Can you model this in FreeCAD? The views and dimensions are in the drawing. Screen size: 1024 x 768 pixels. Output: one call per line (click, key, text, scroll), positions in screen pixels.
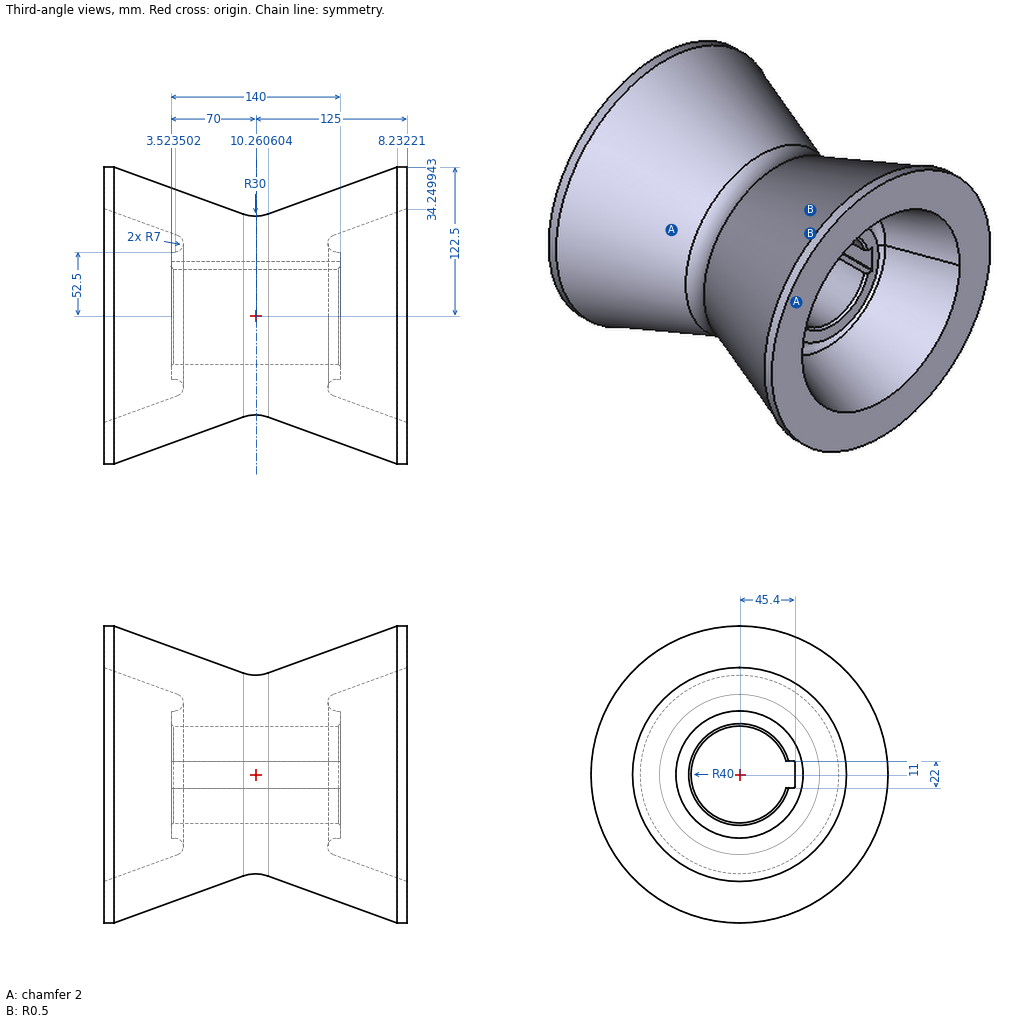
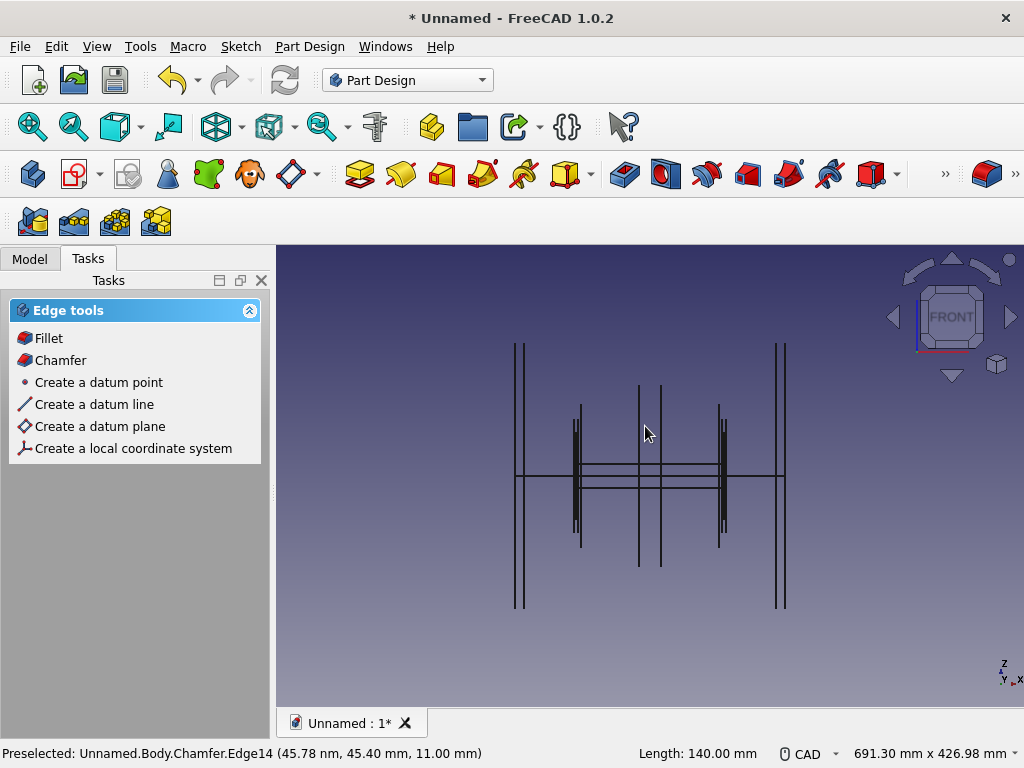
key(3)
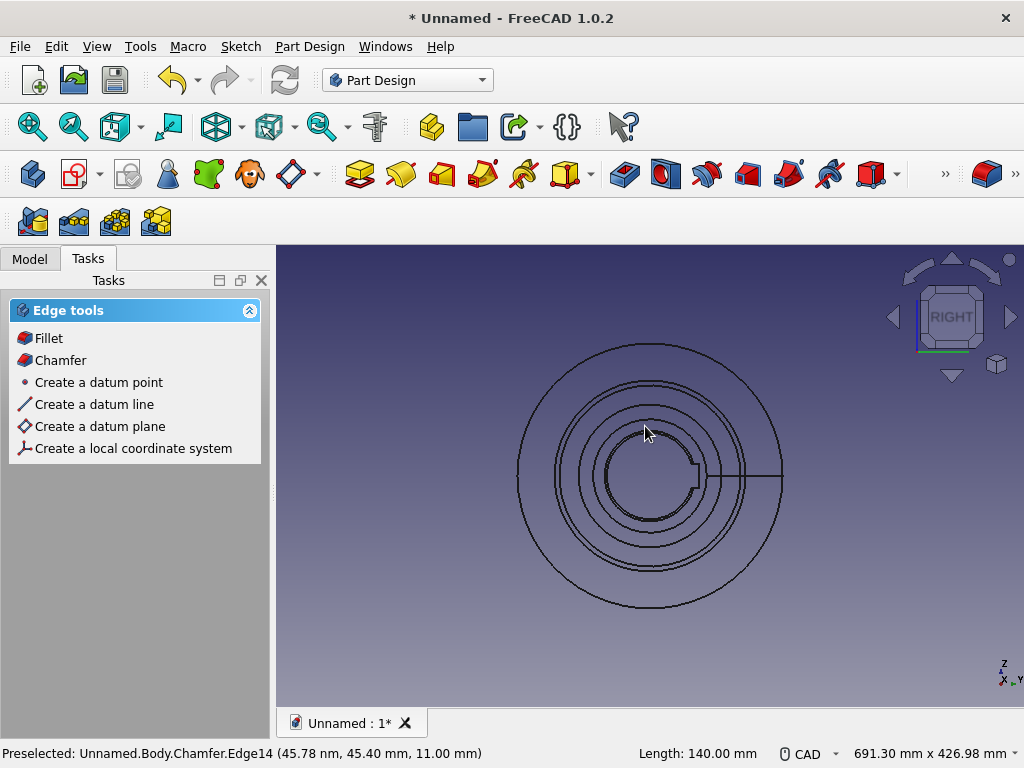
key(5)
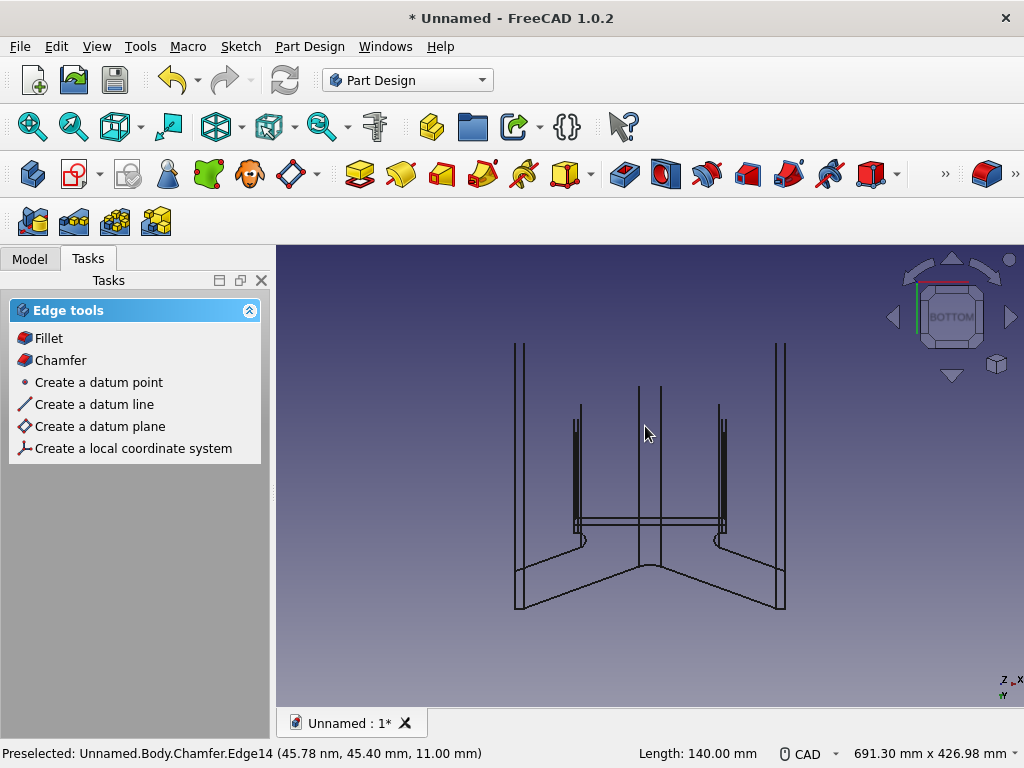
click(650, 524, ctrl)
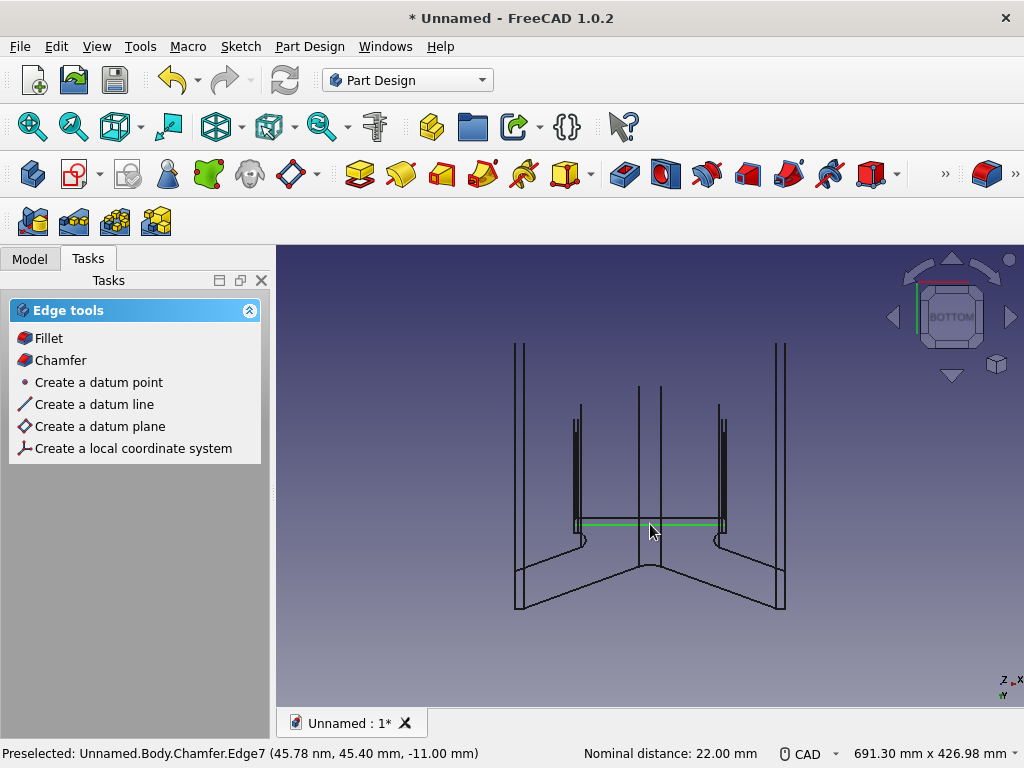
key(v)
key(1)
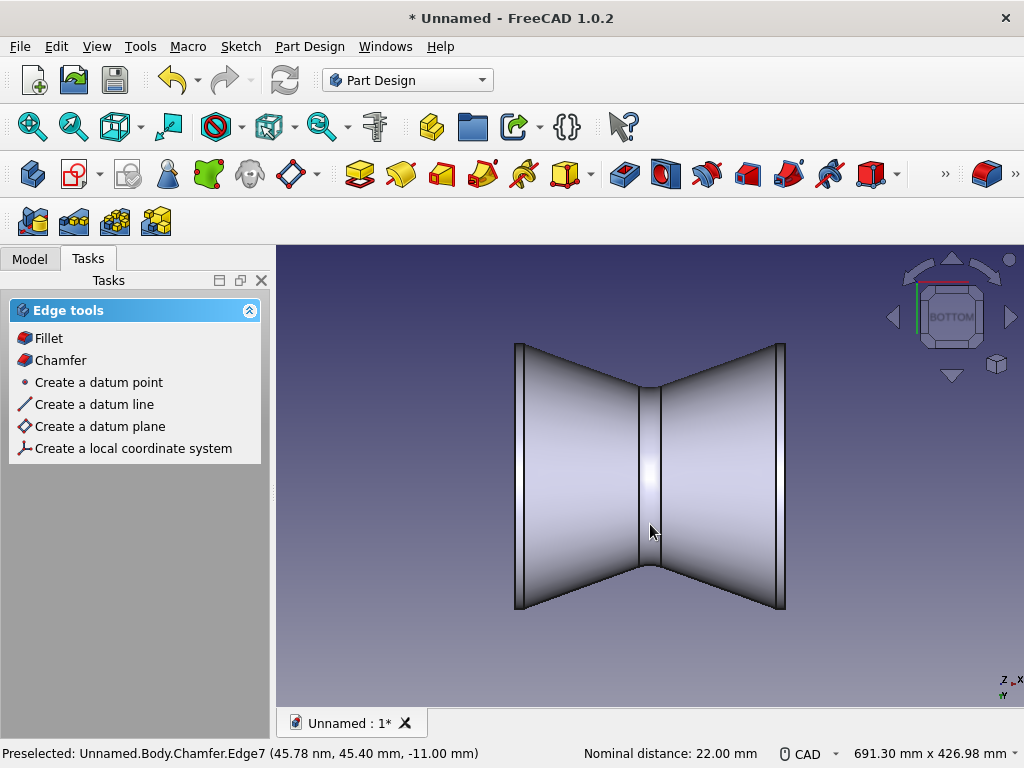
click(987, 174)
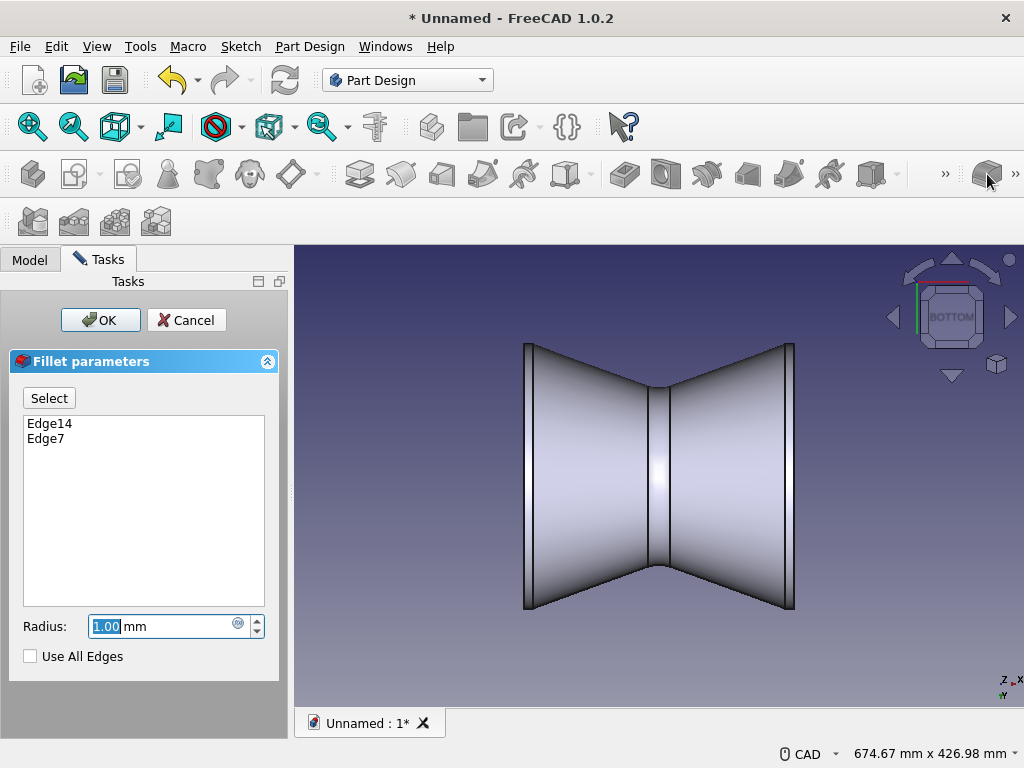
text(0.5)
key(Tab)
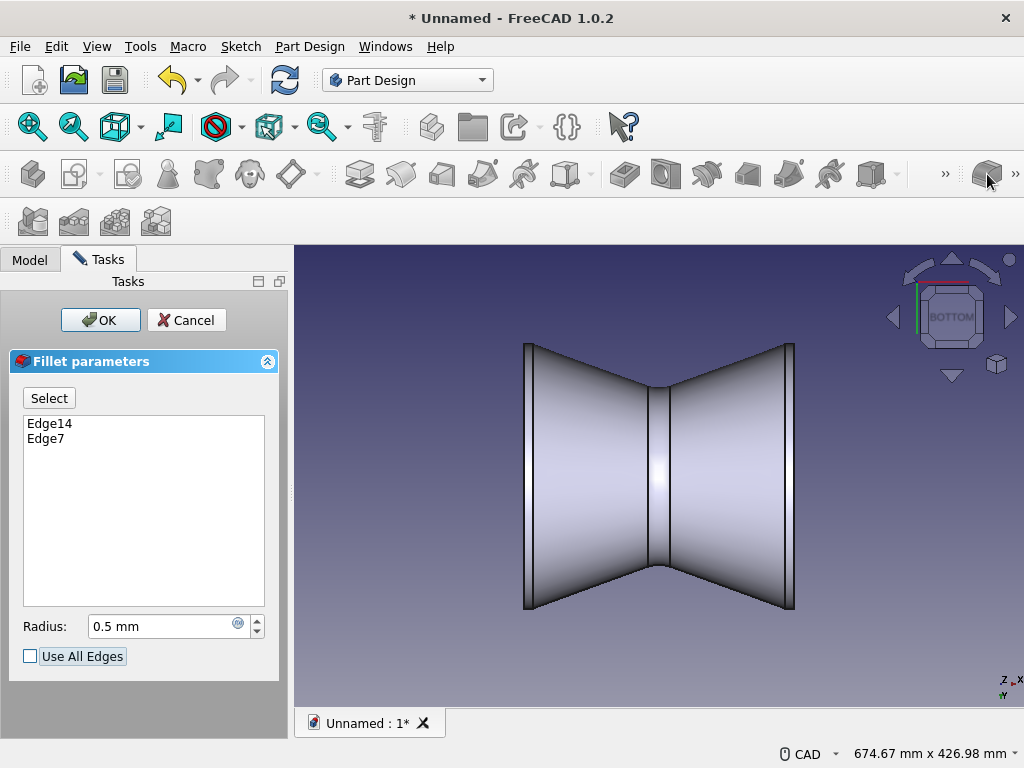
click(101, 320)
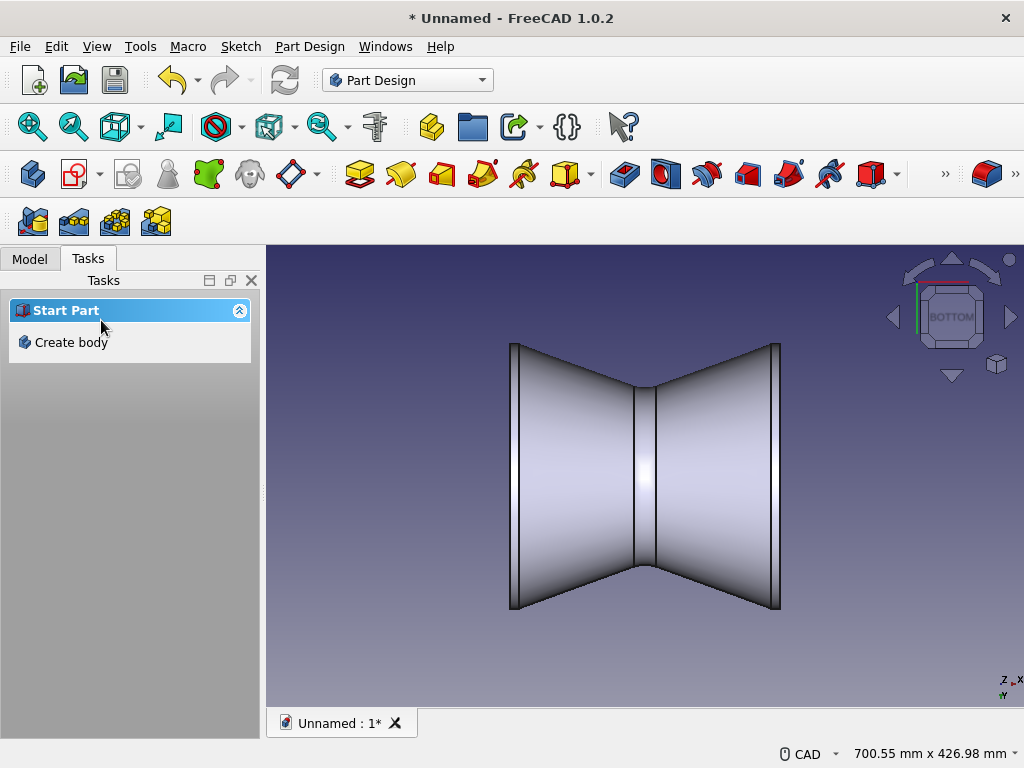
key(0)